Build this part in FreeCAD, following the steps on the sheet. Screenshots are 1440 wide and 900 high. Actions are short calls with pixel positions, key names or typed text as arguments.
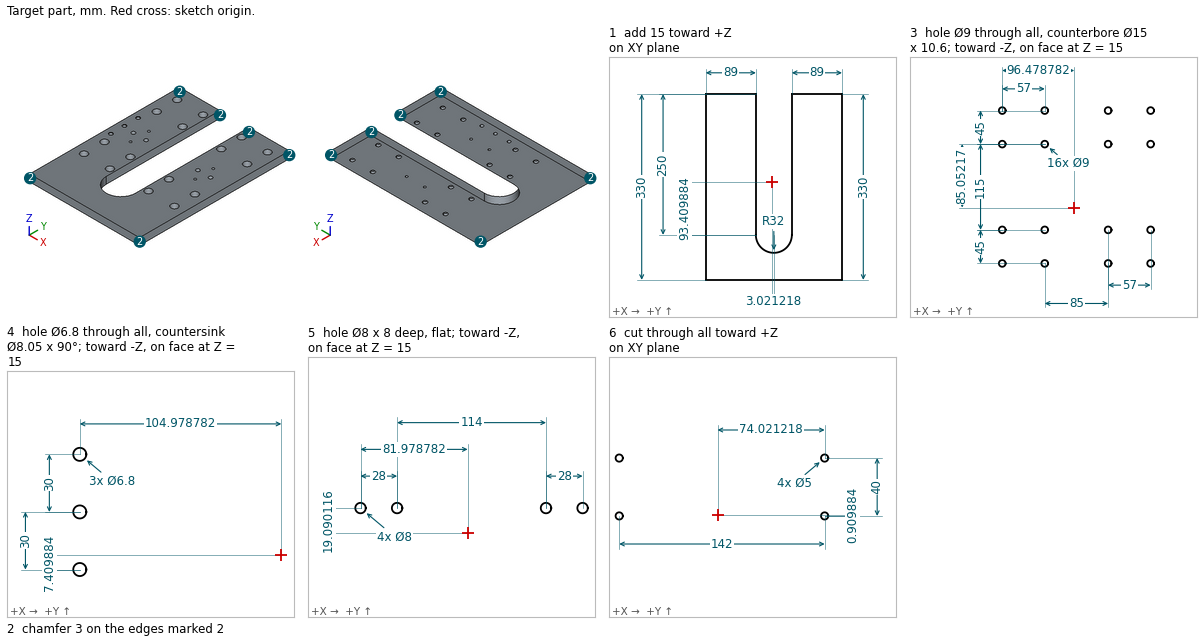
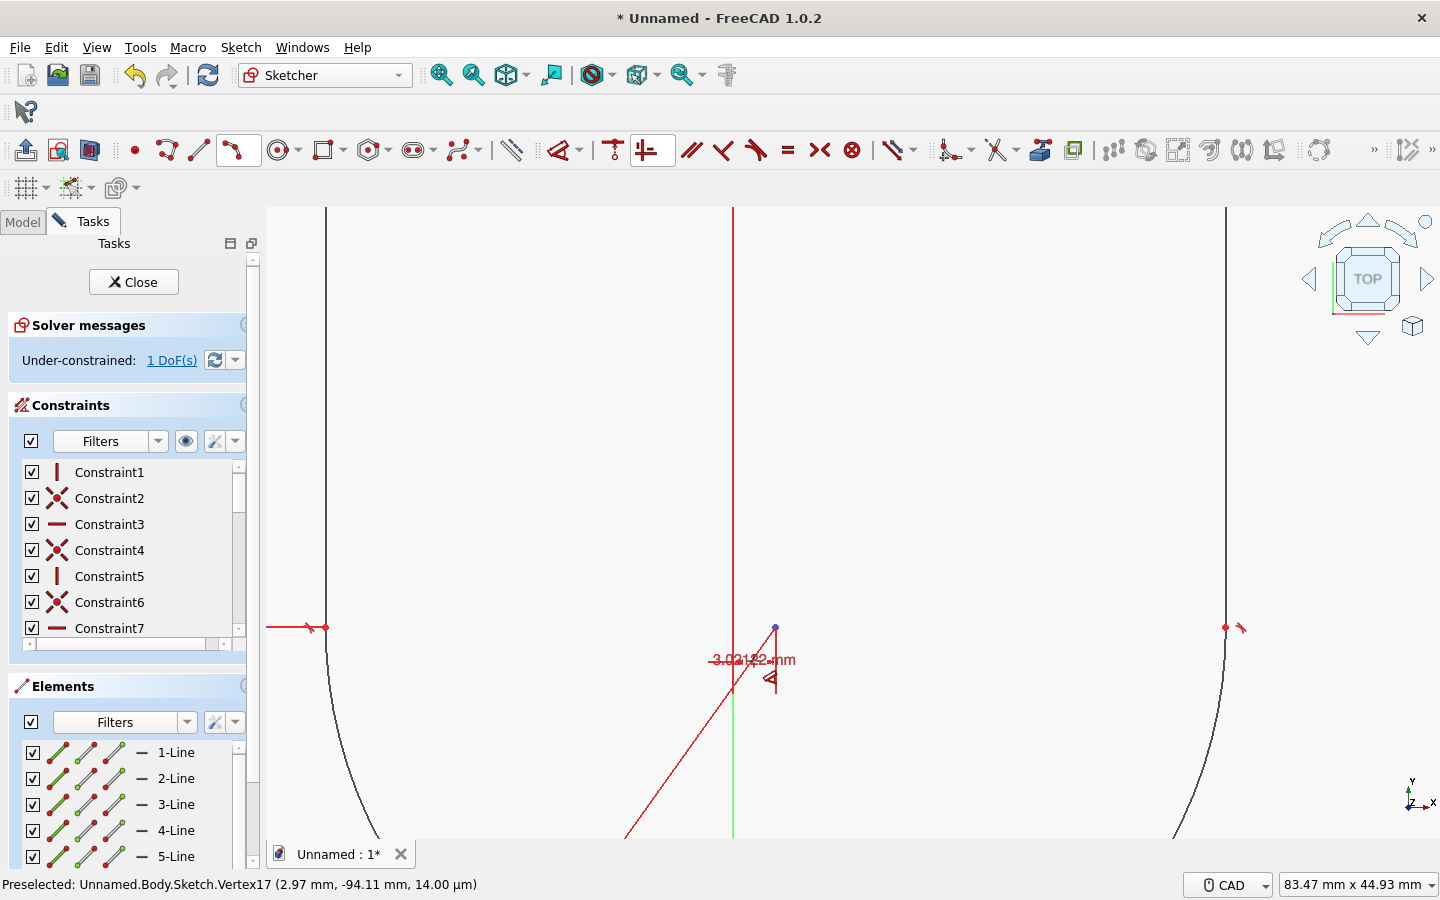
scroll(785, 633, down, 12)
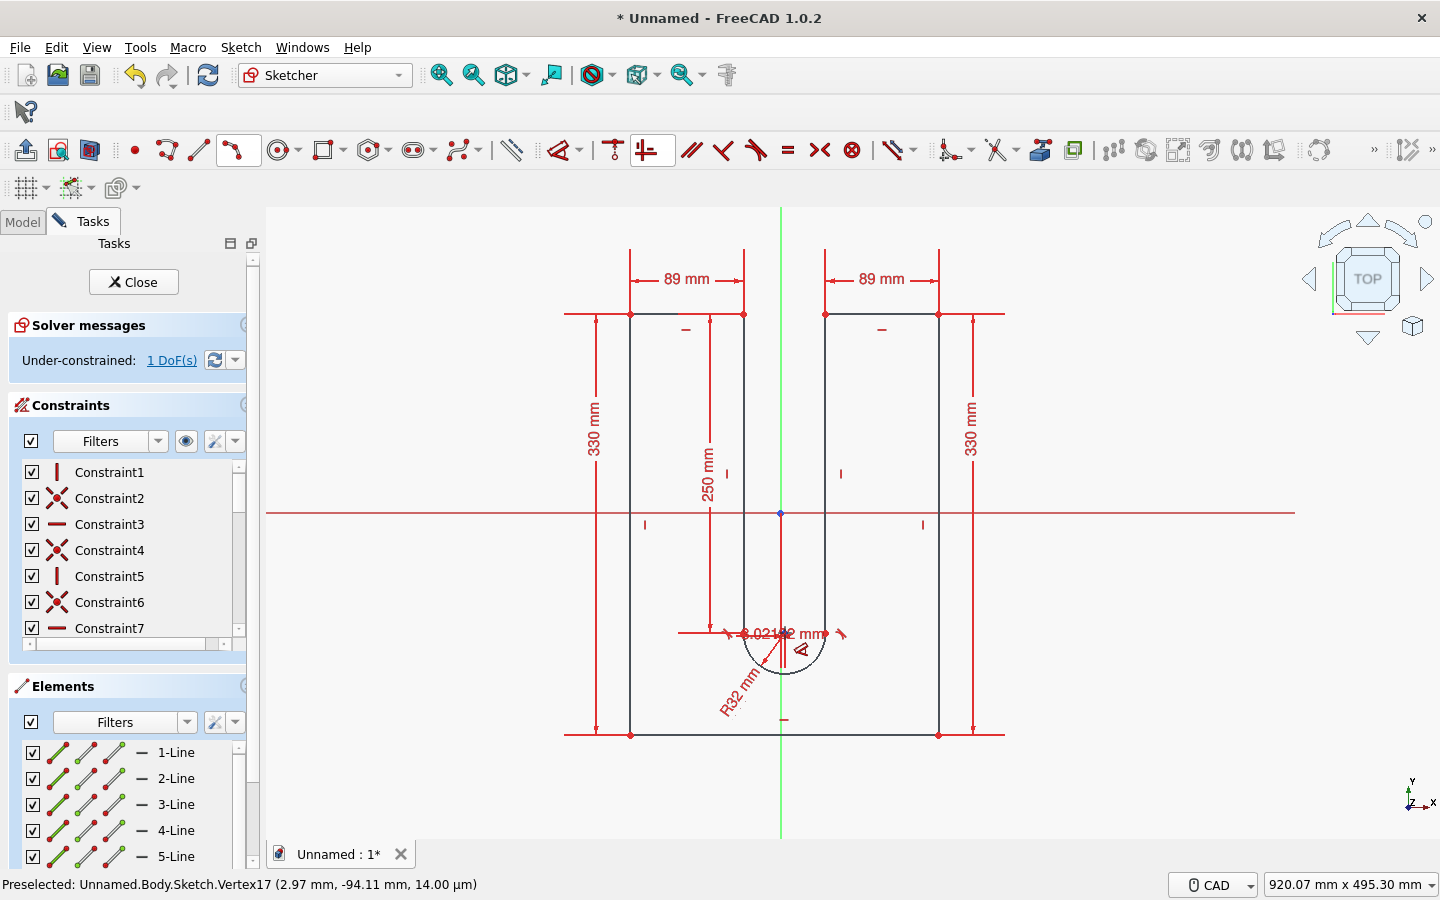
click(744, 633)
click(710, 573)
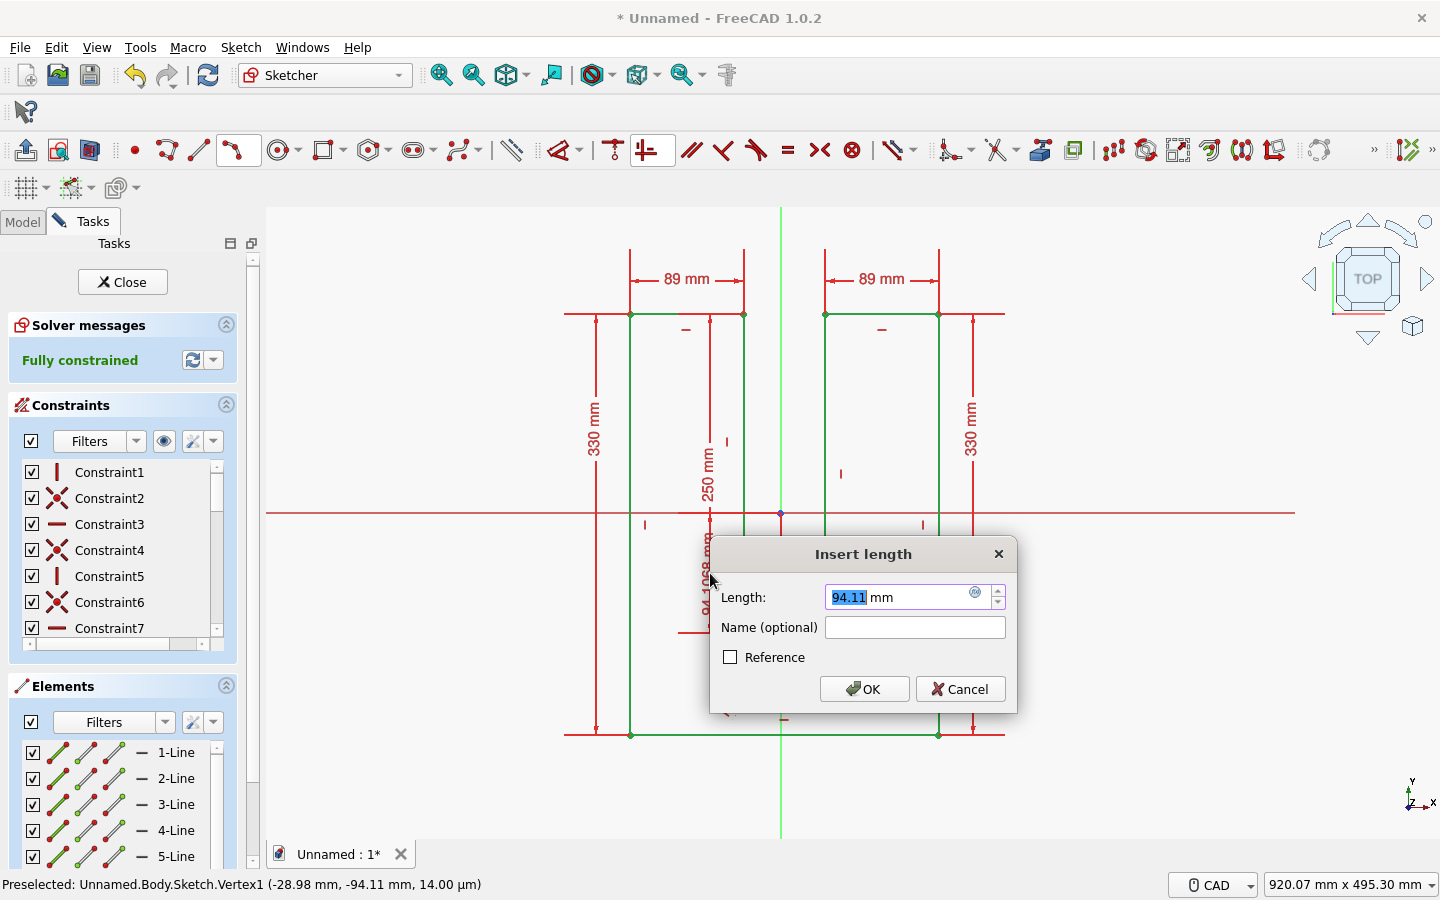
text(93.409884)
key(Return)
key(Escape)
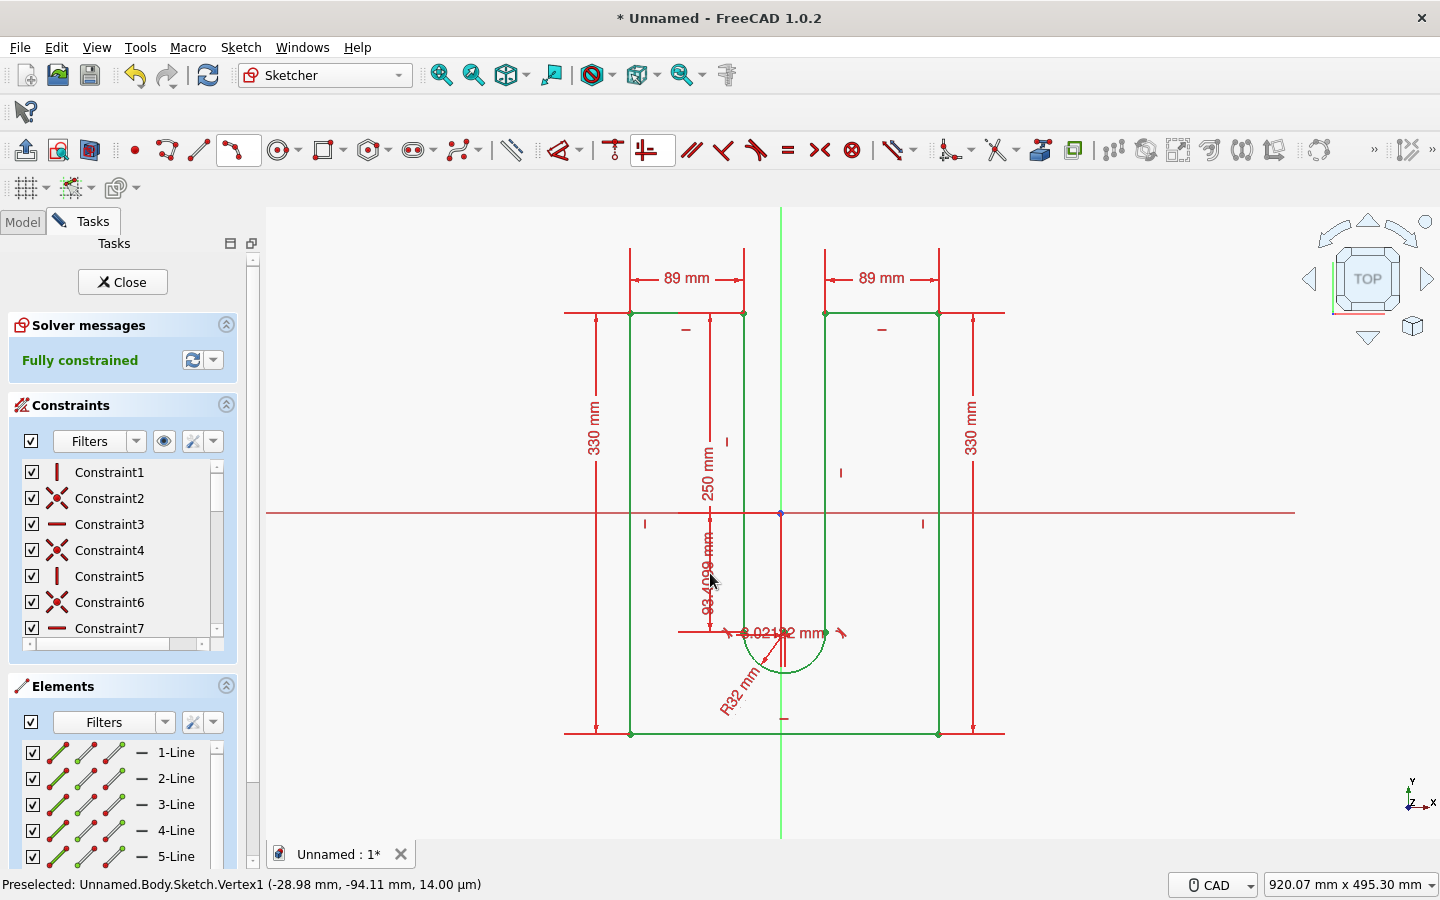
click(123, 282)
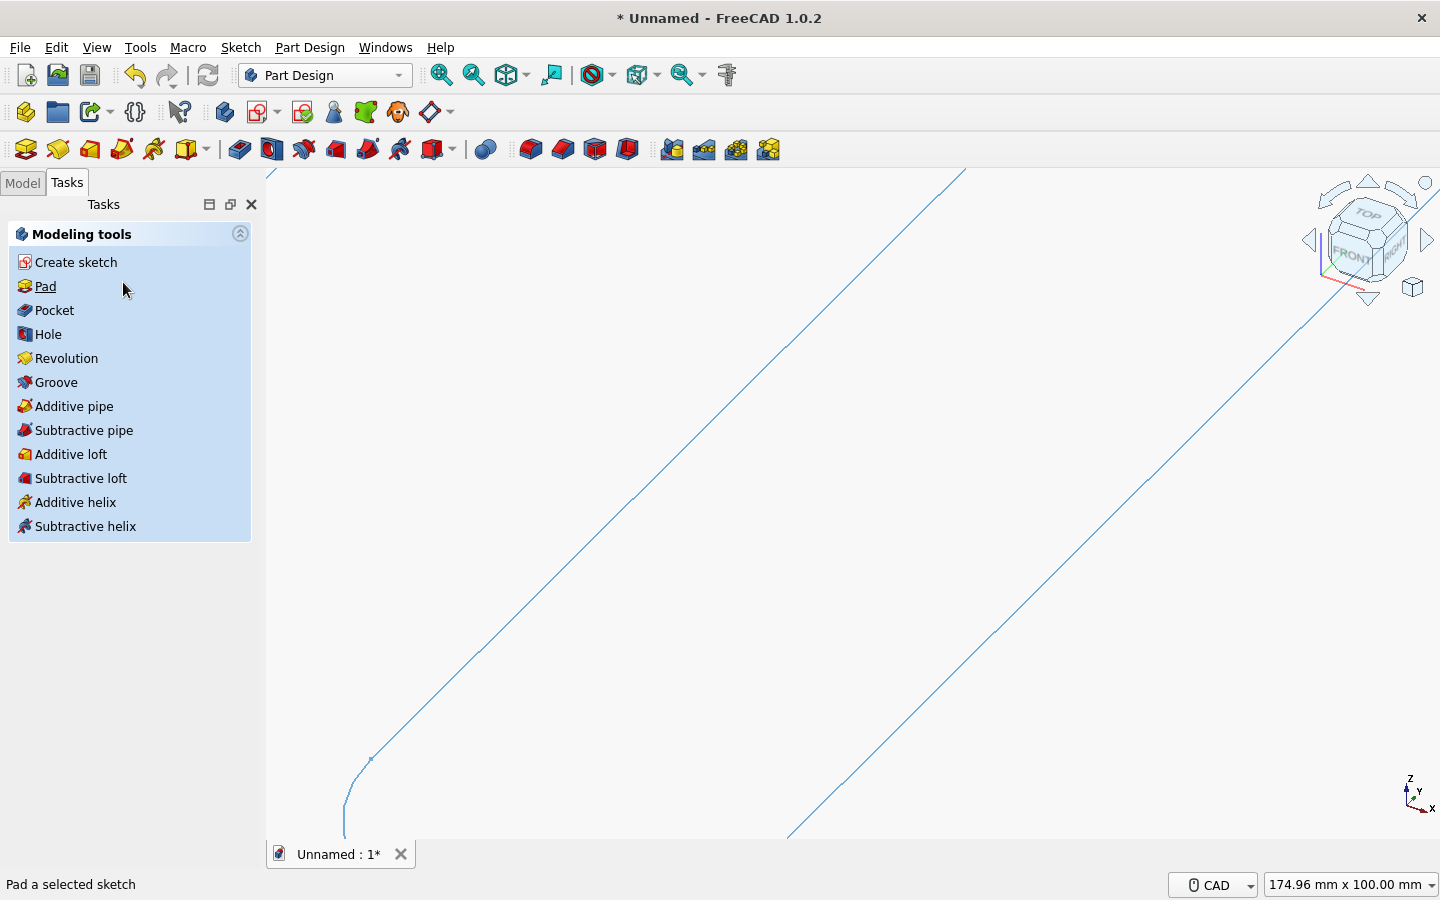
click(26, 150)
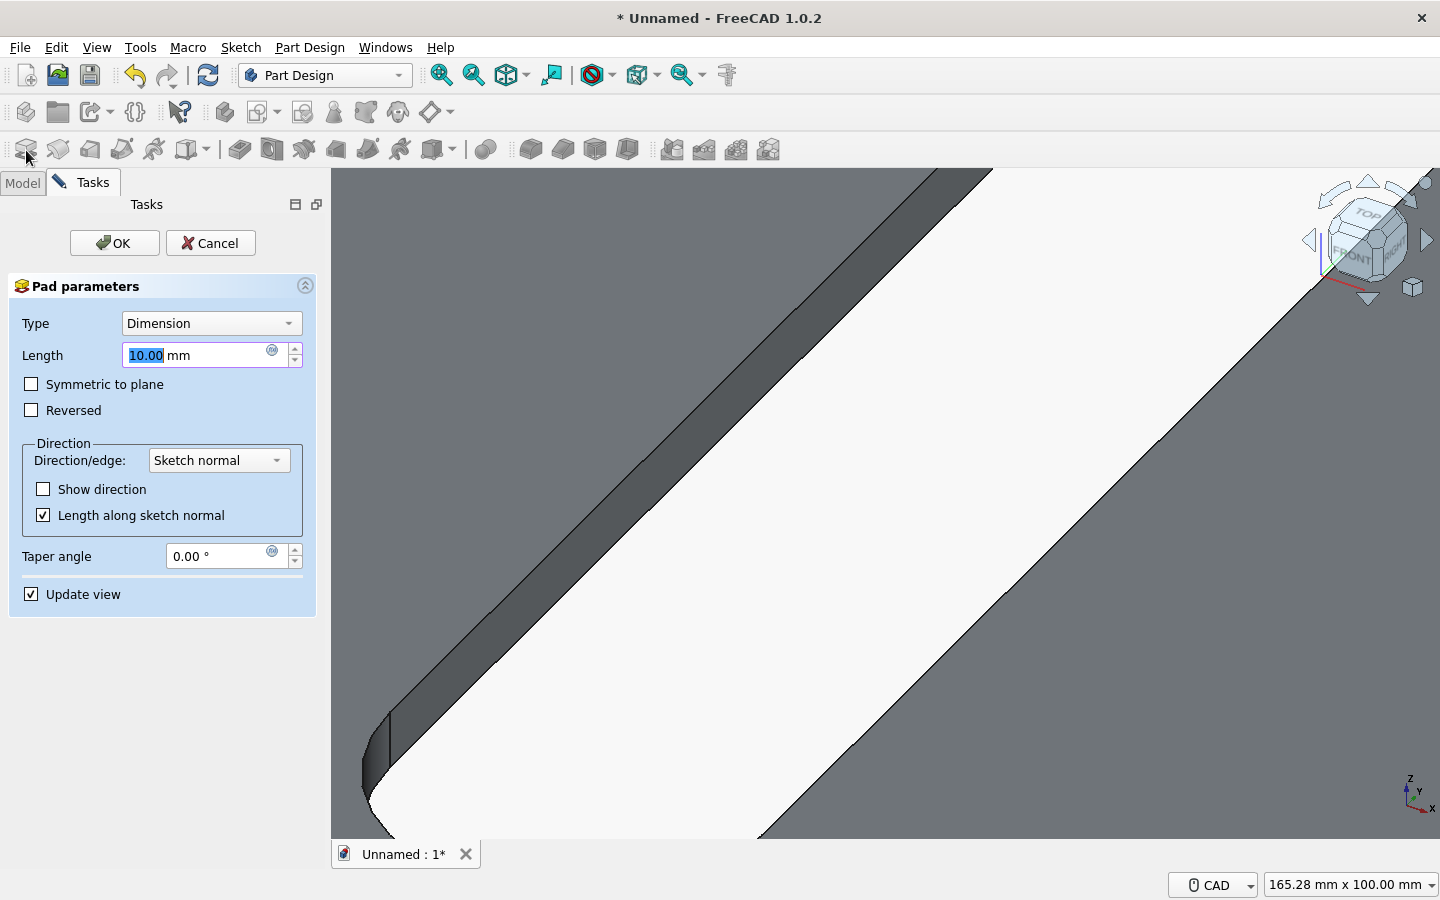
text(15)
key(Tab)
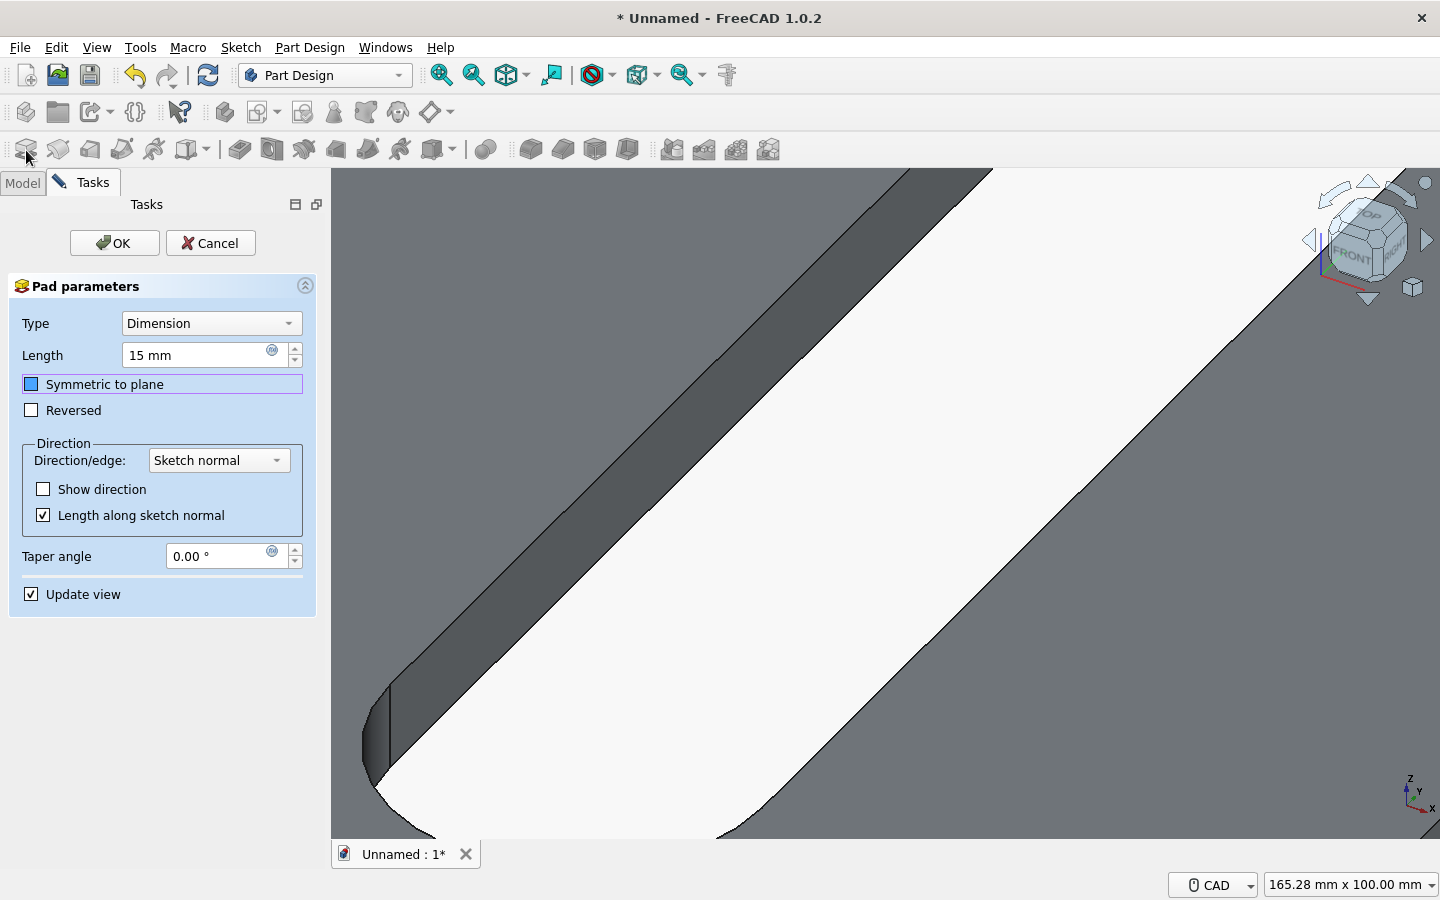
click(115, 243)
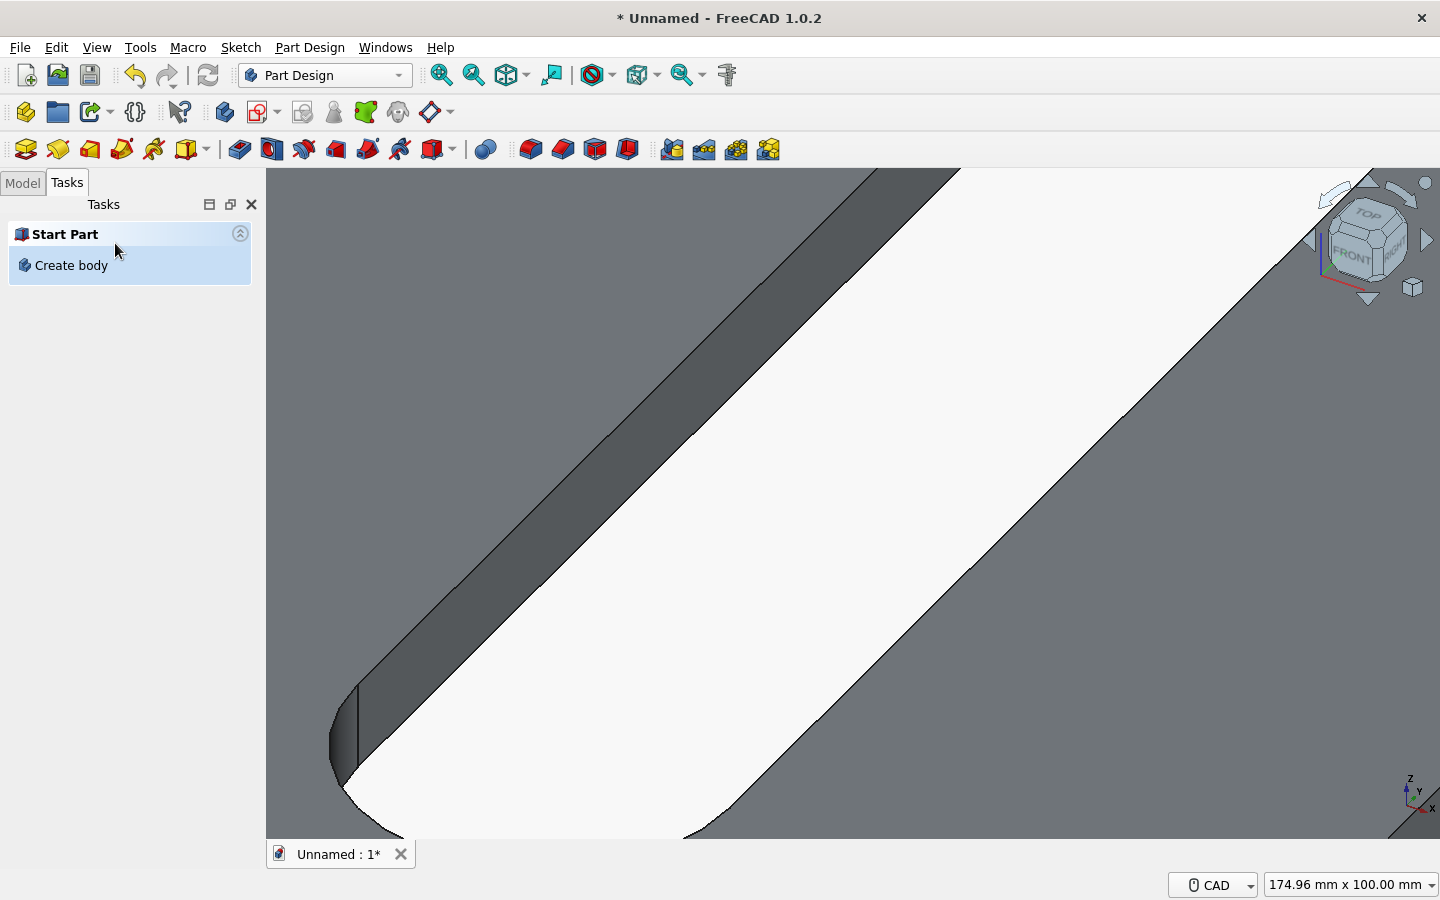
key(v)
key(f)